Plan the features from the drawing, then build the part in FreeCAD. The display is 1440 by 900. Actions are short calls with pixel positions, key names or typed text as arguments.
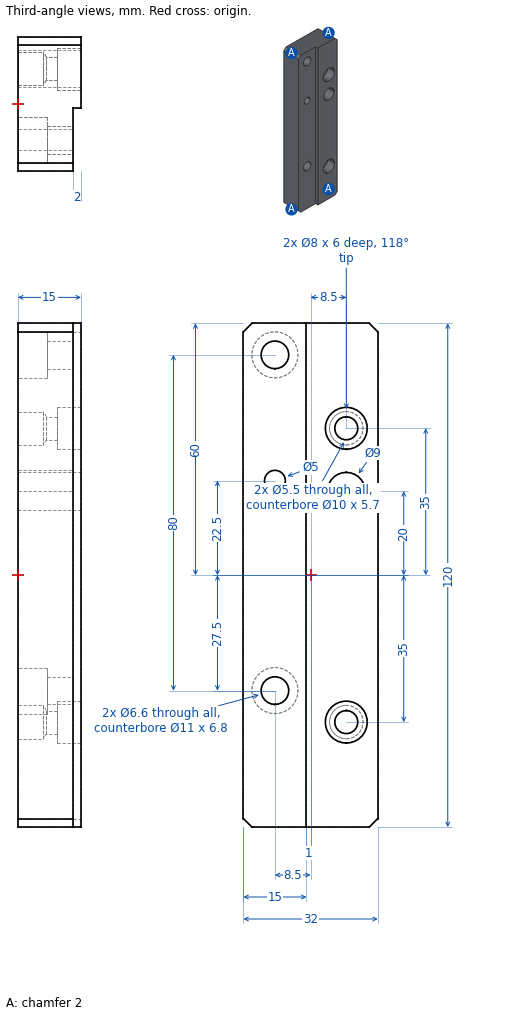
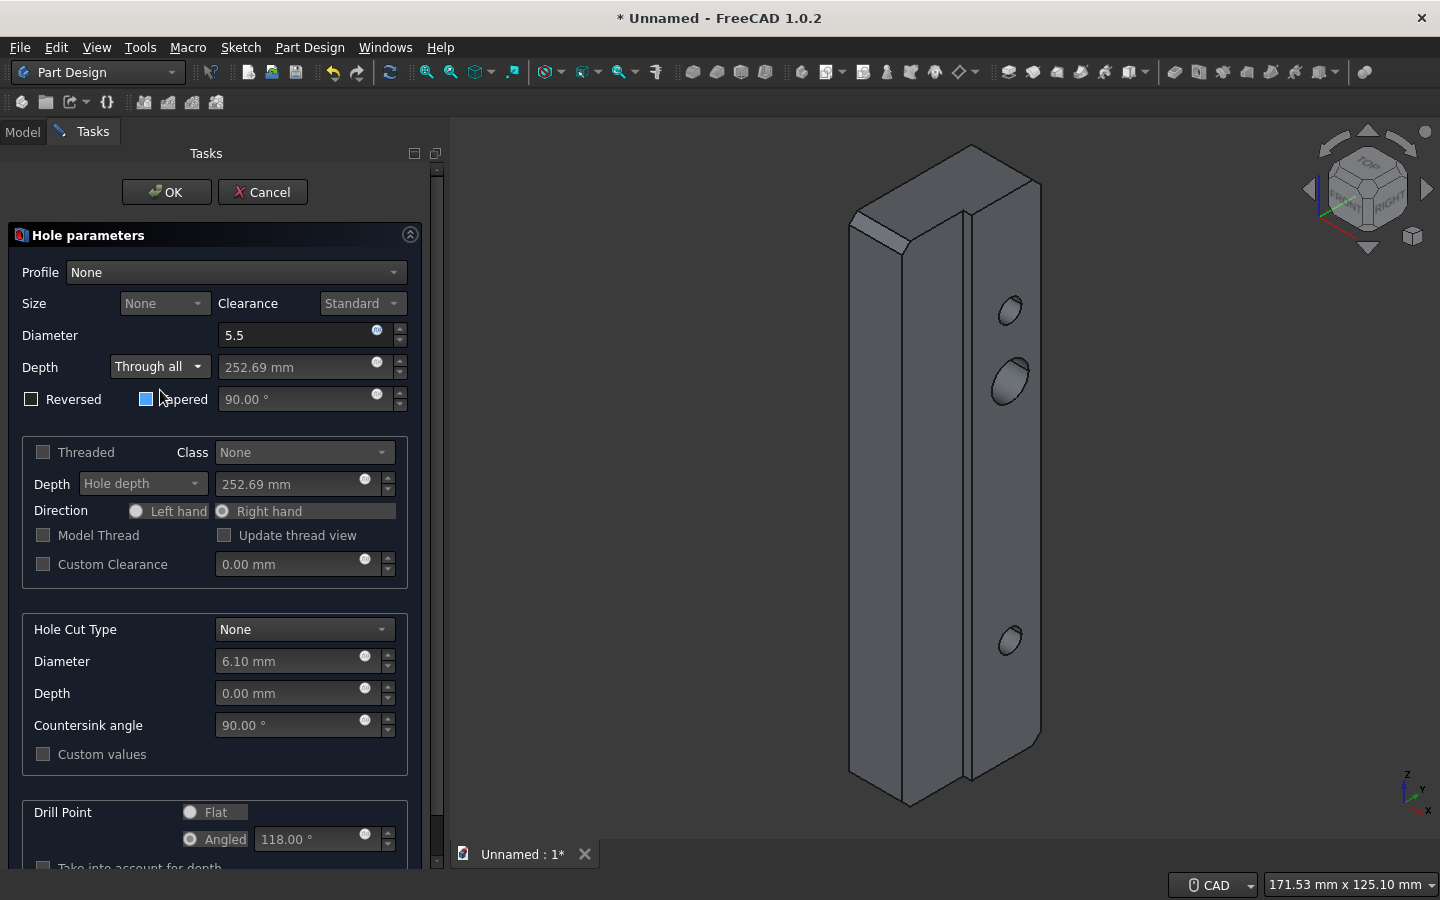
click(306, 630)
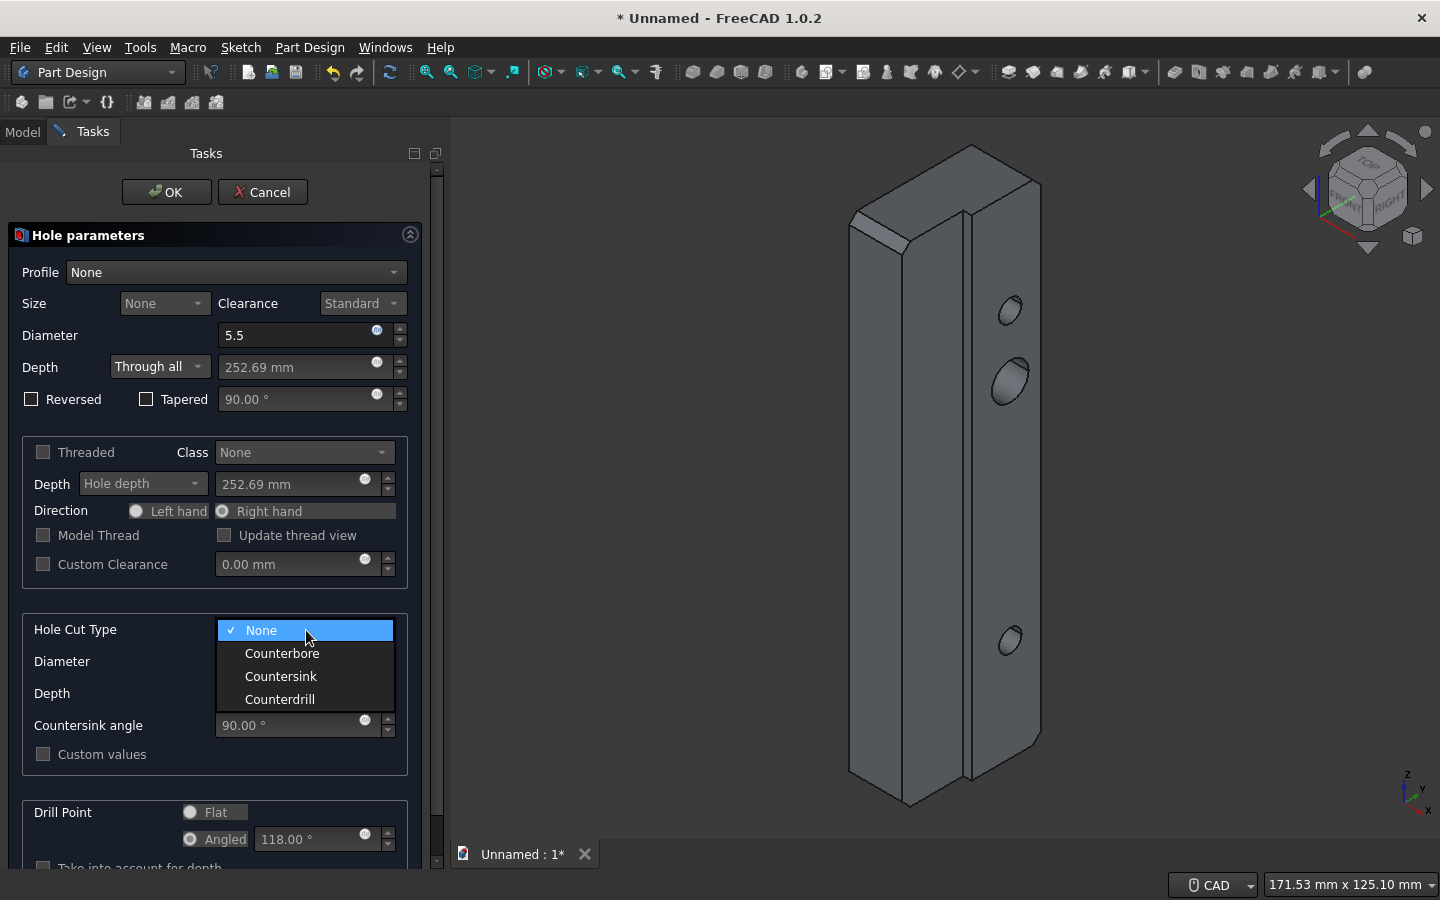
click(304, 654)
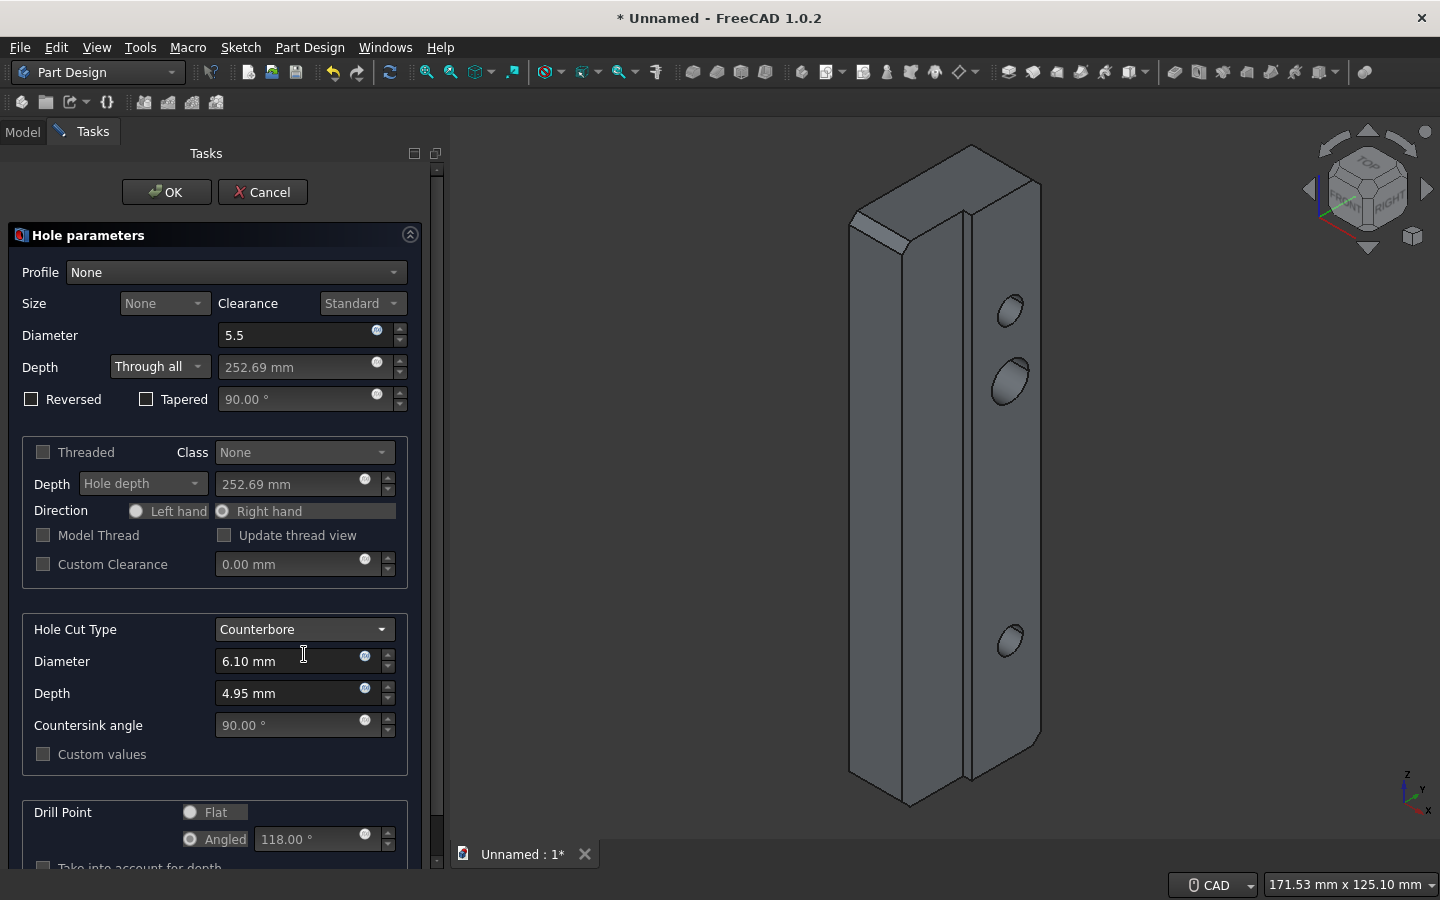
triple_click(298, 661)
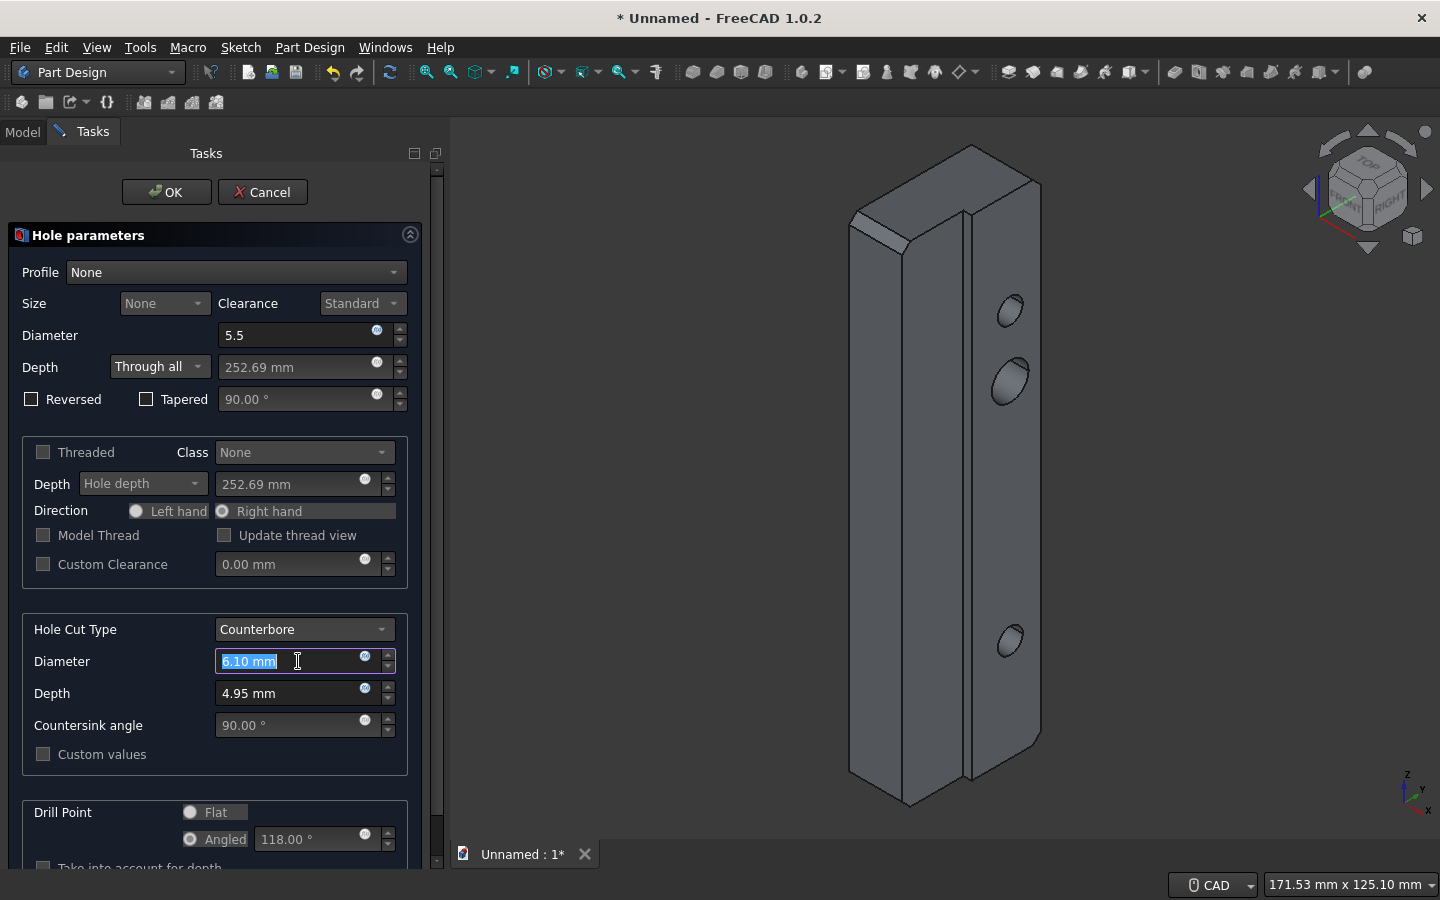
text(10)
key(Tab)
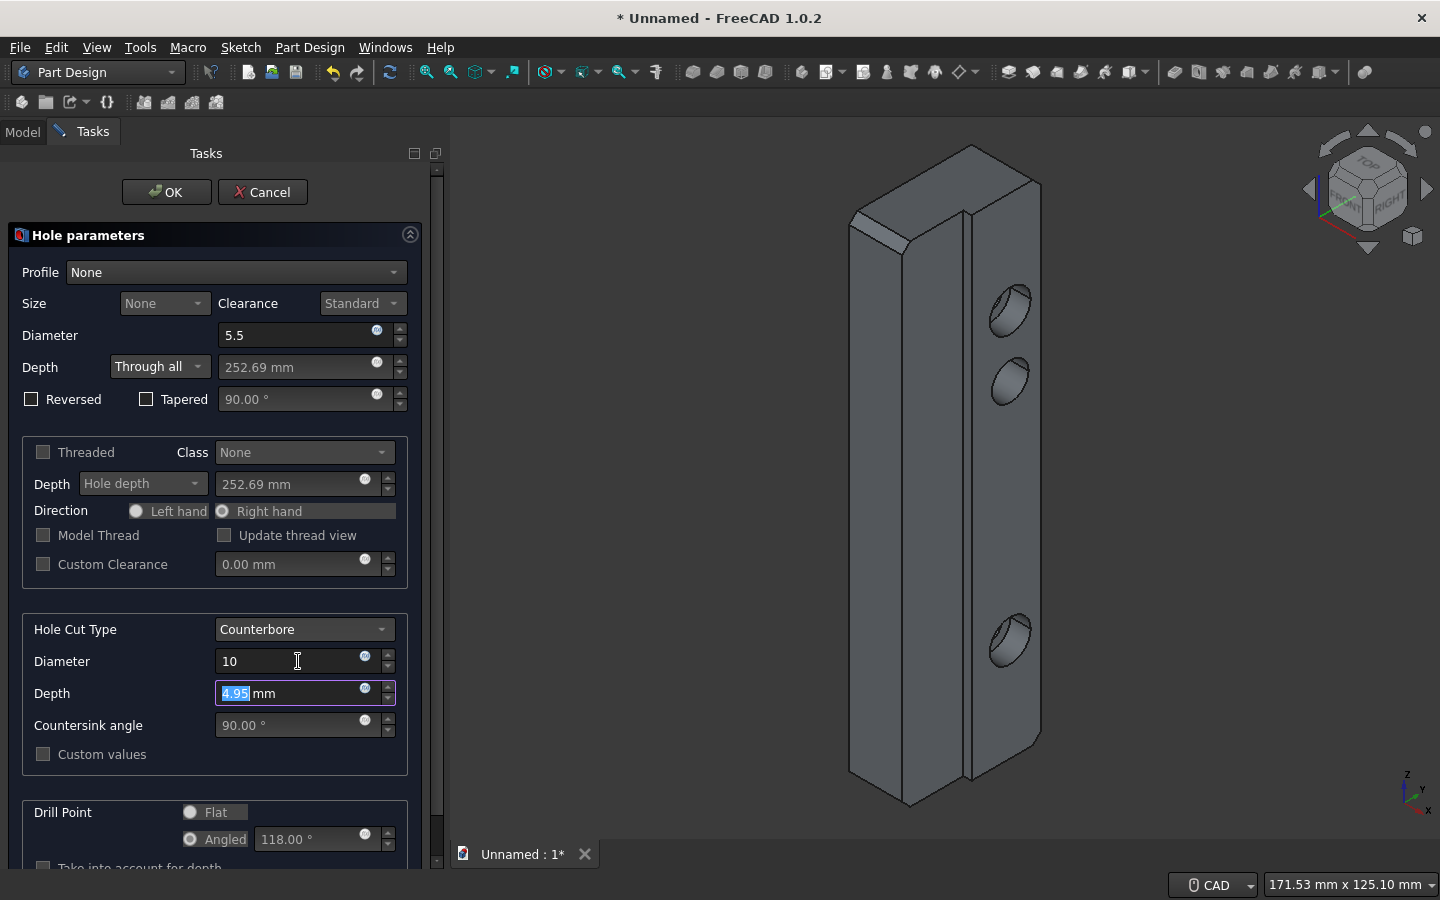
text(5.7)
key(Tab)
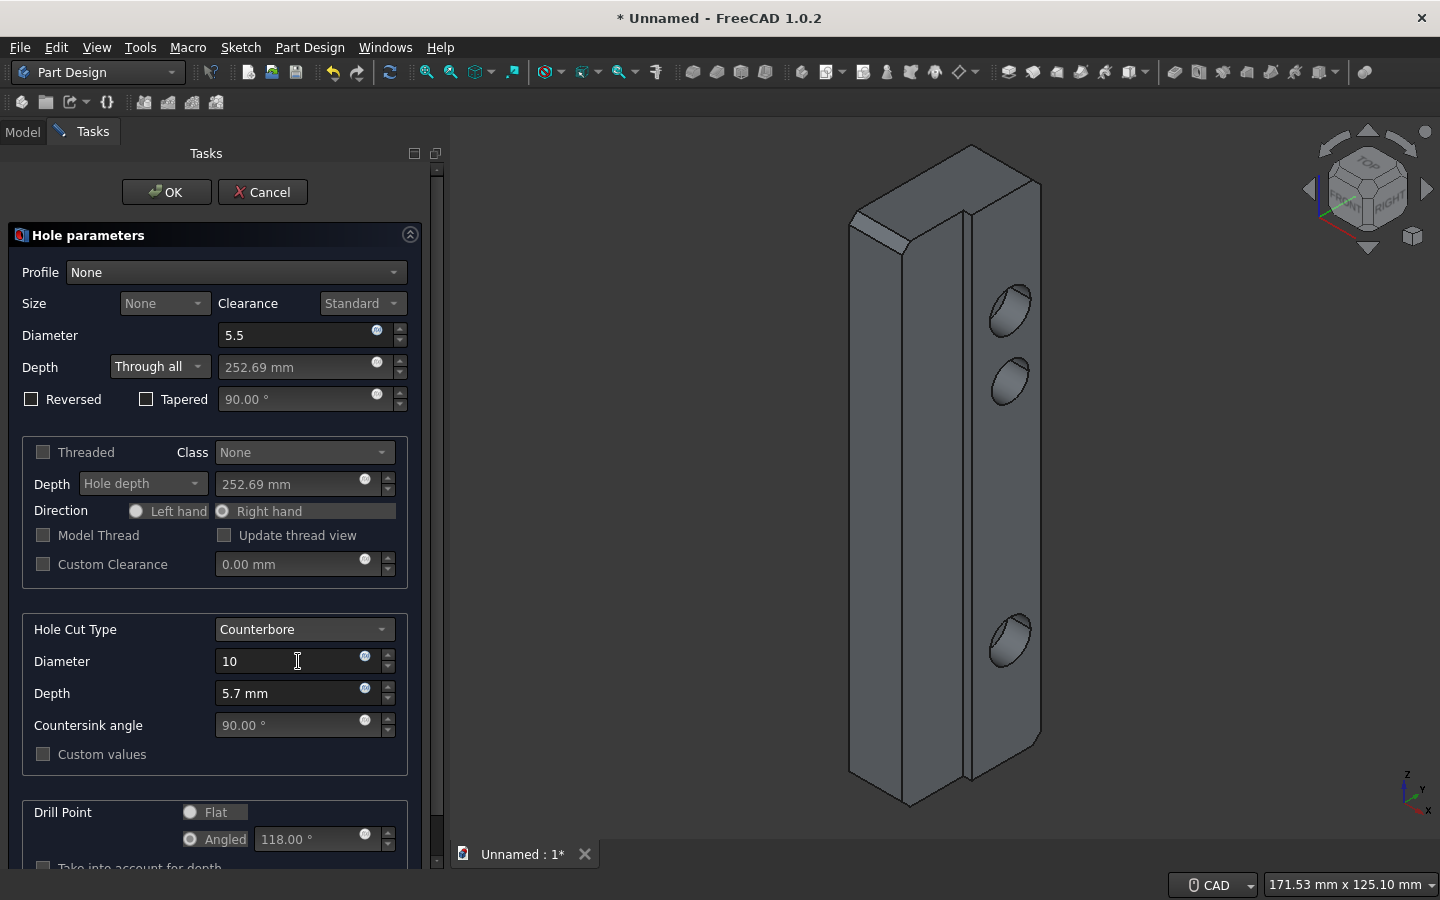
click(167, 192)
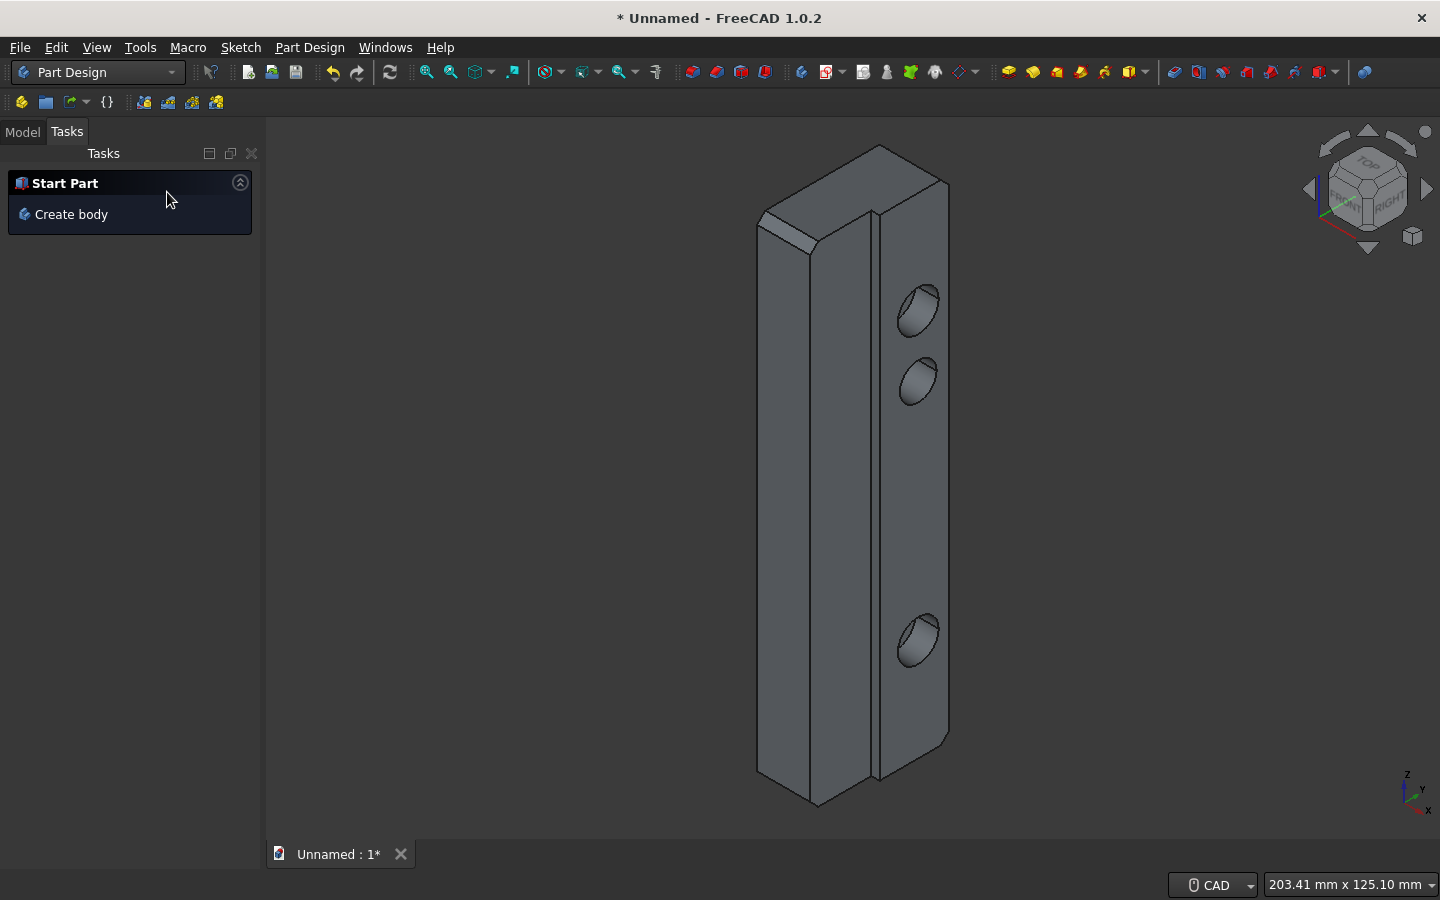
click(826, 72)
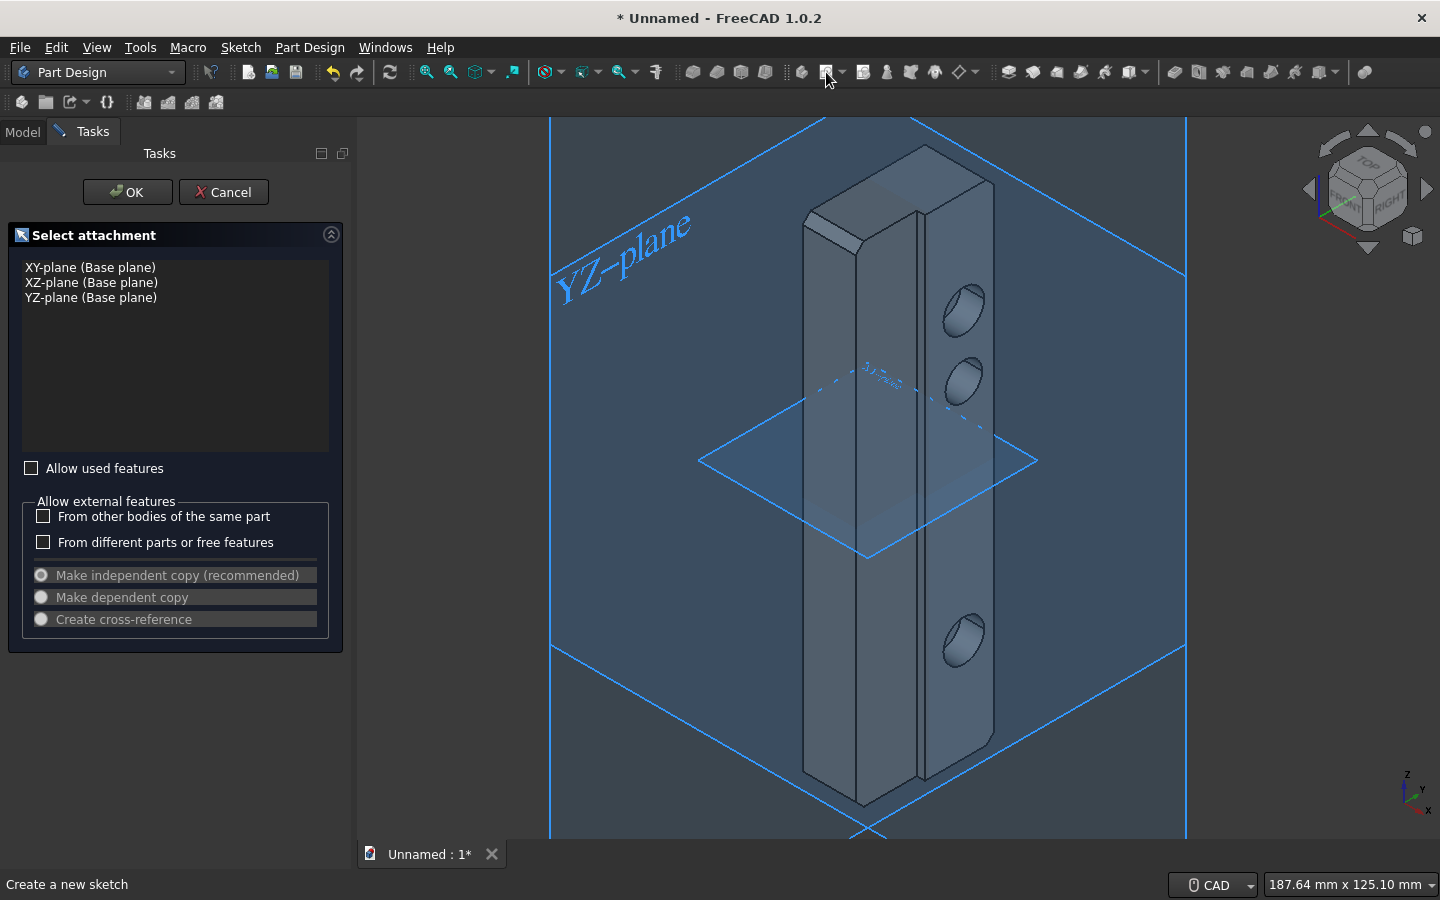
click(82, 298)